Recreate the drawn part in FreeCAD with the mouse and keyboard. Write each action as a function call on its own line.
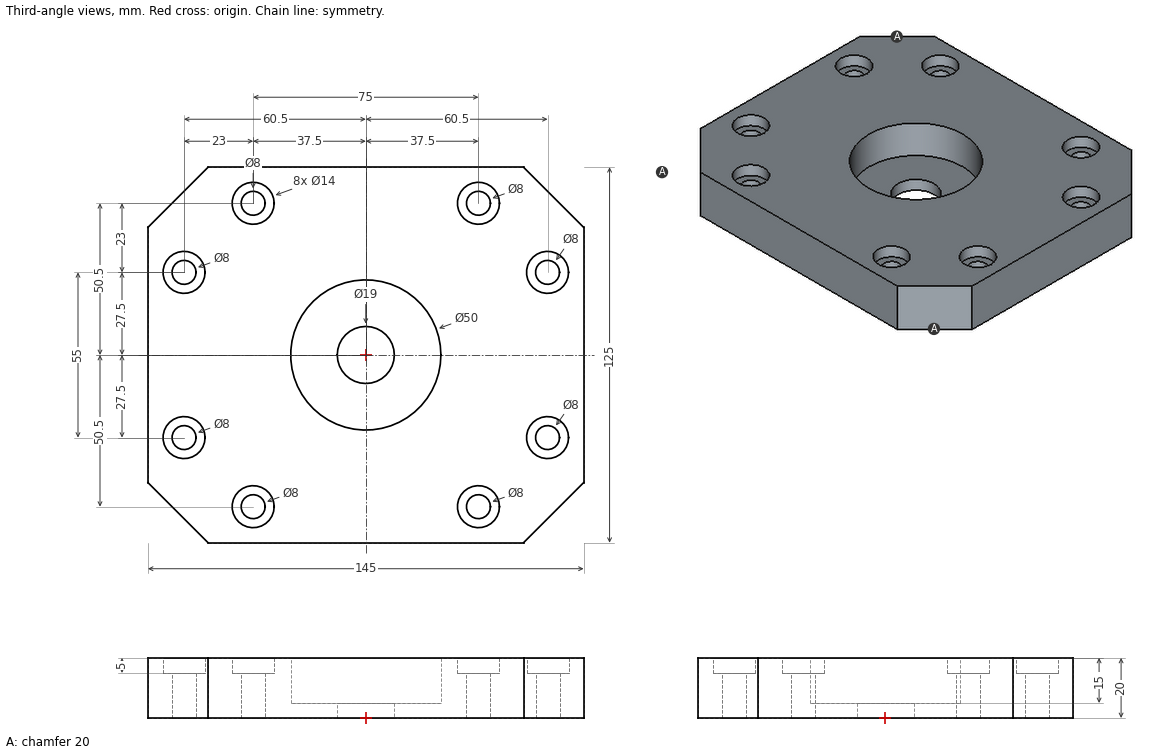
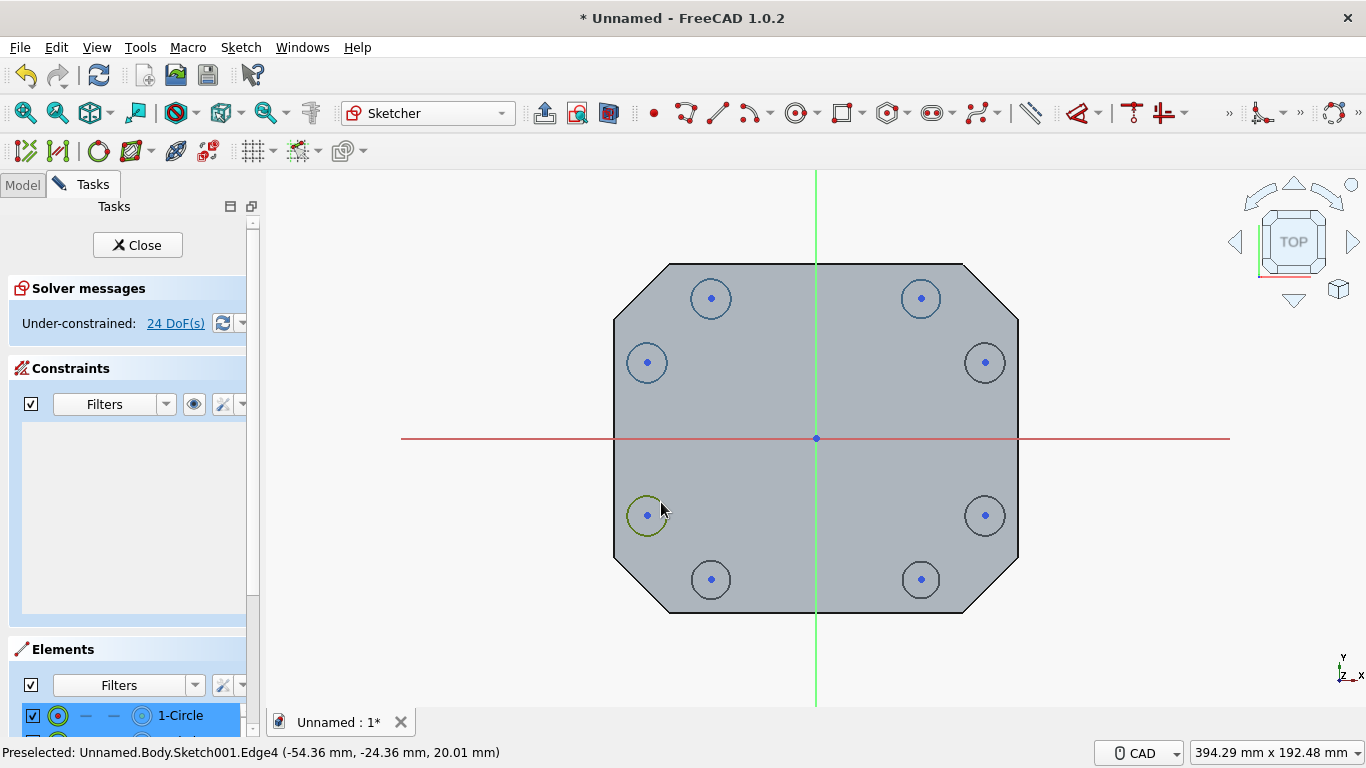
click(724, 566)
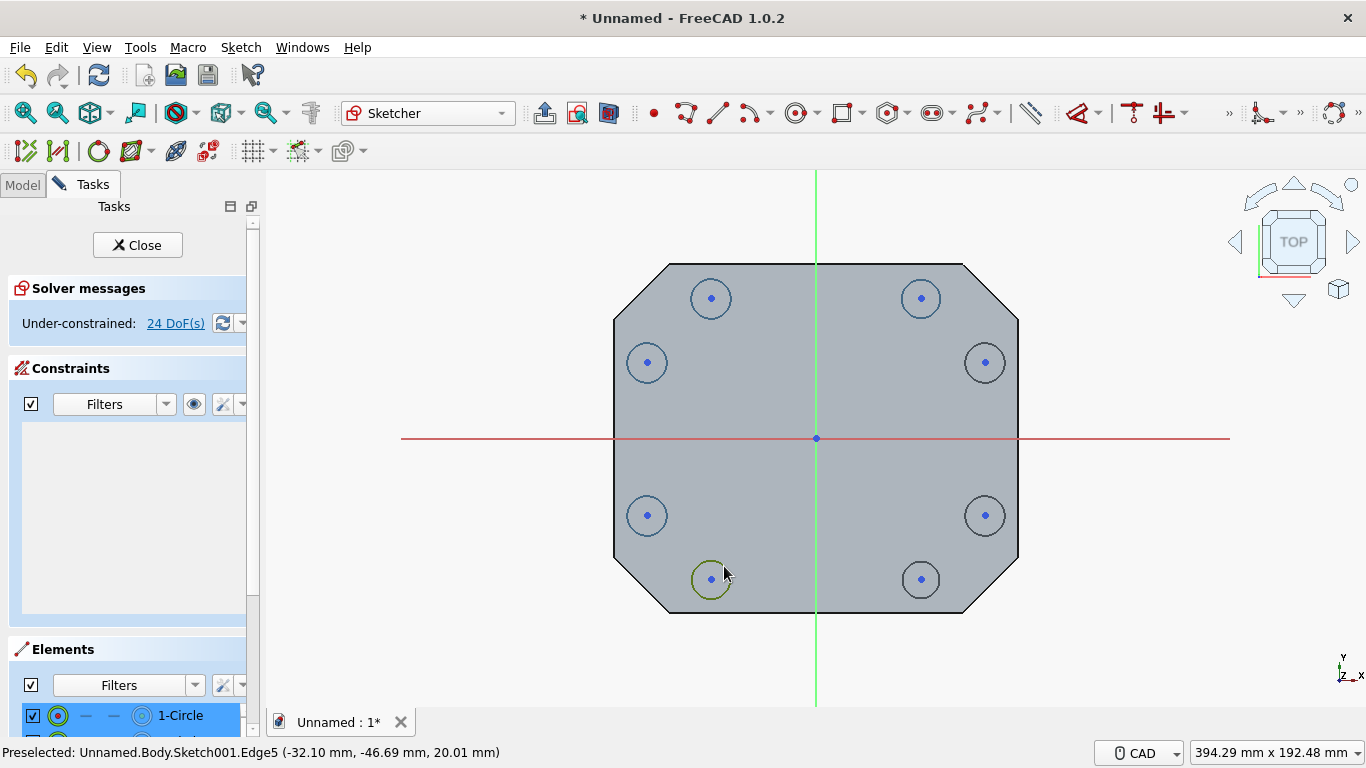
click(934, 567)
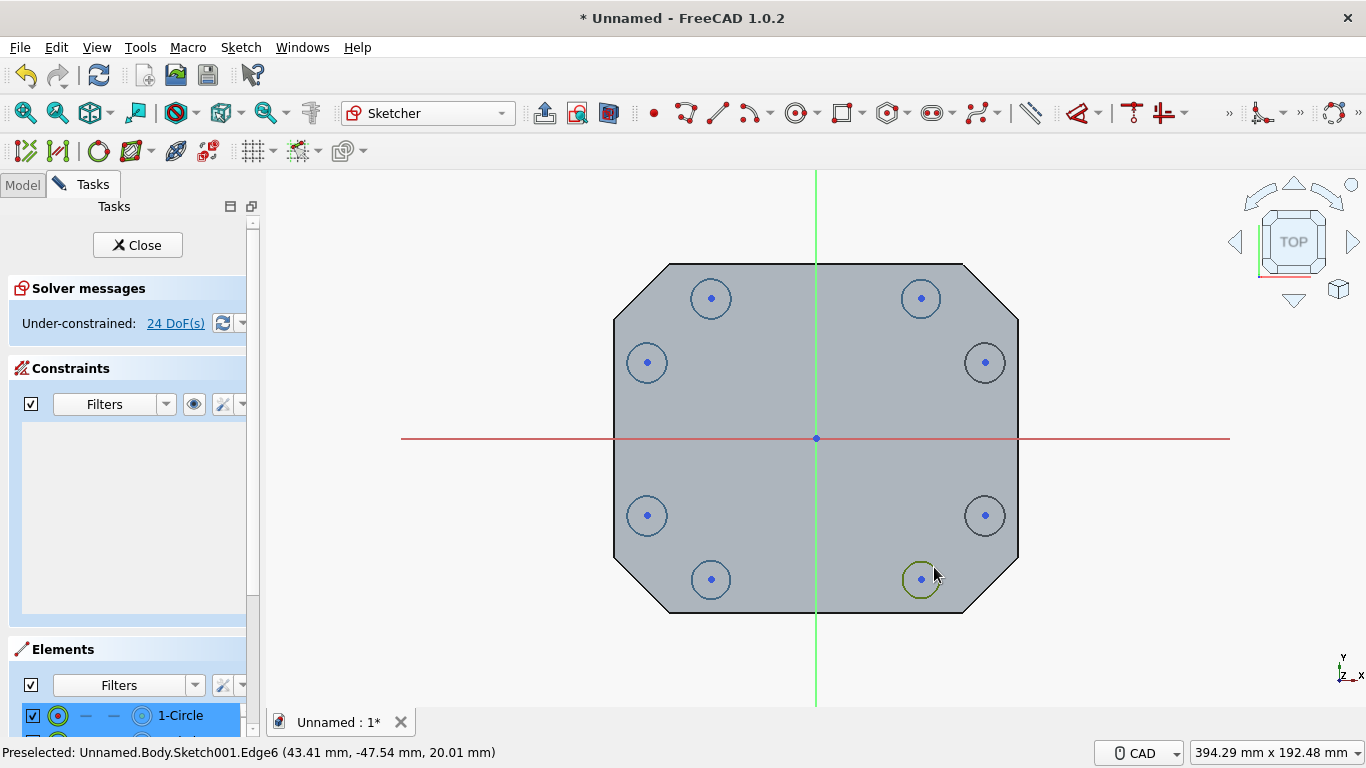
click(999, 349)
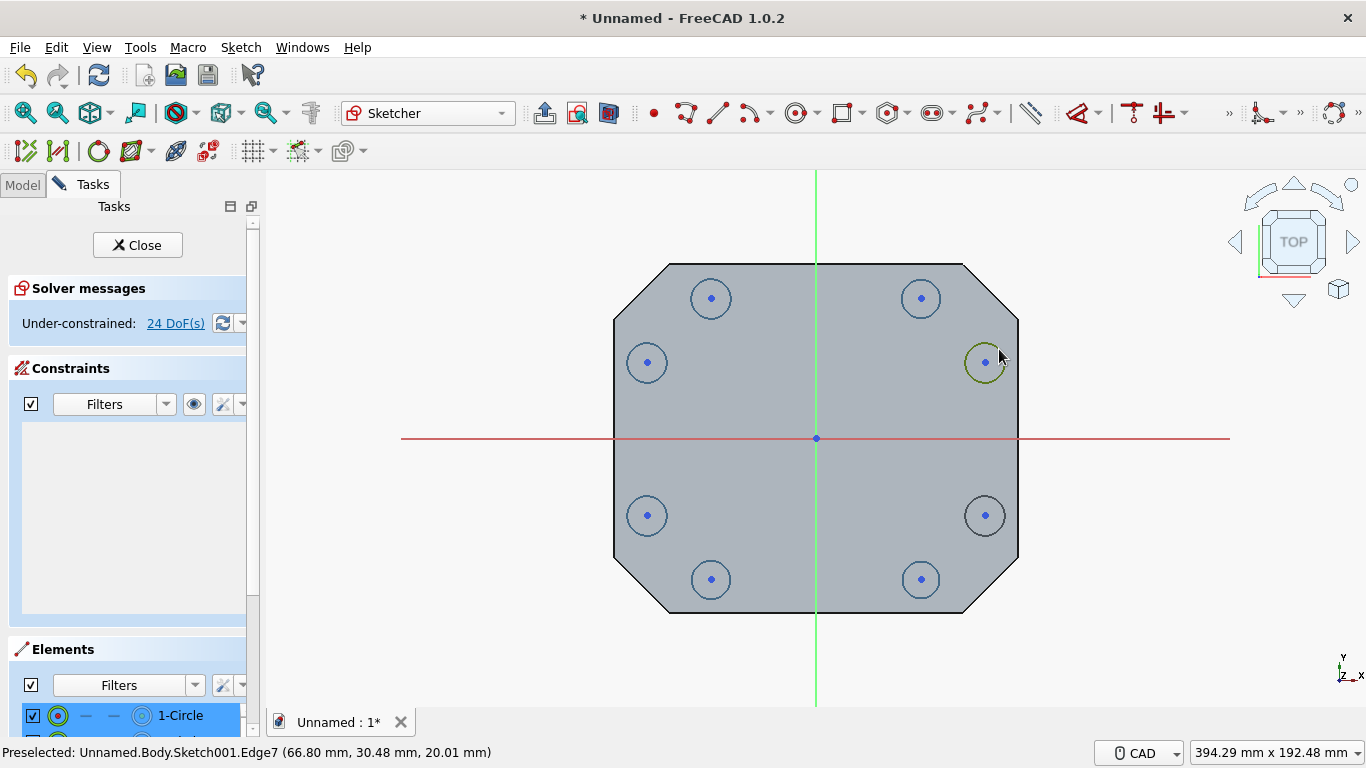
click(999, 502)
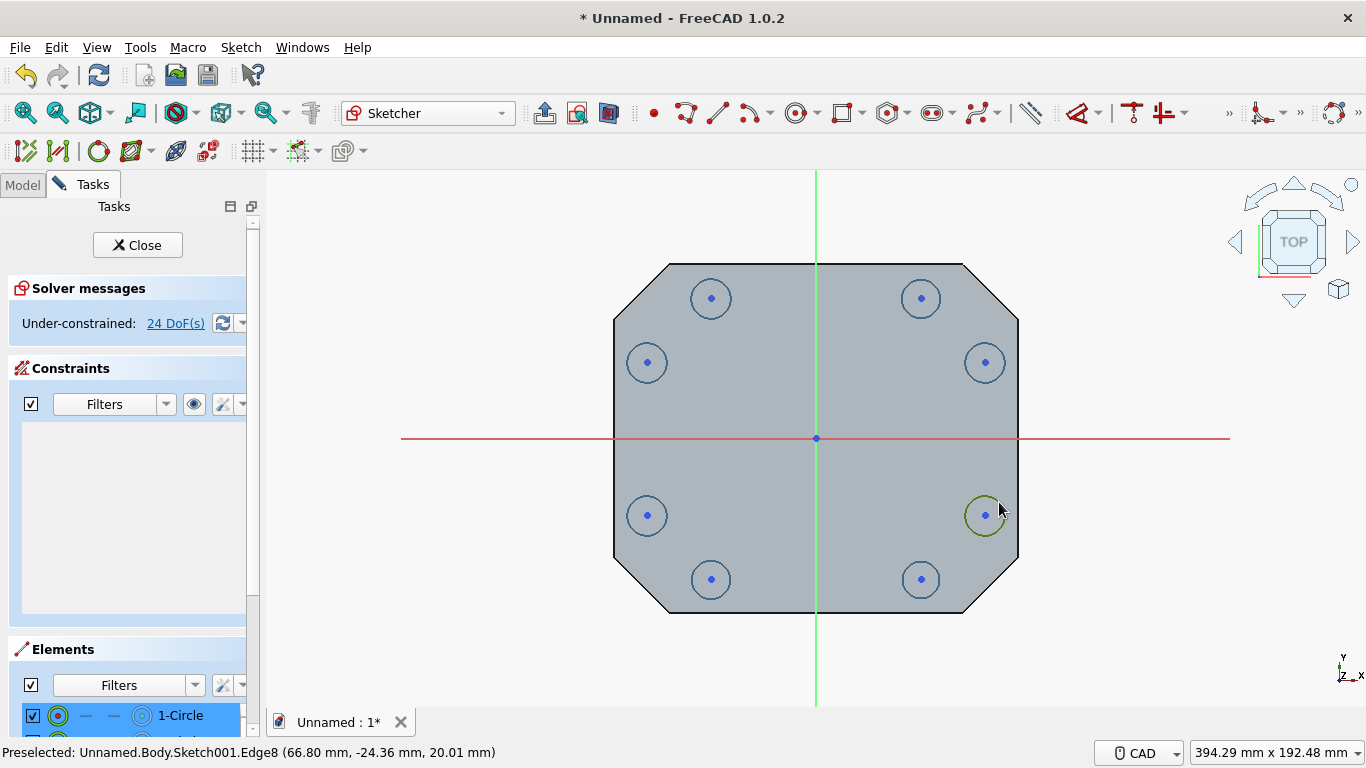
key(e)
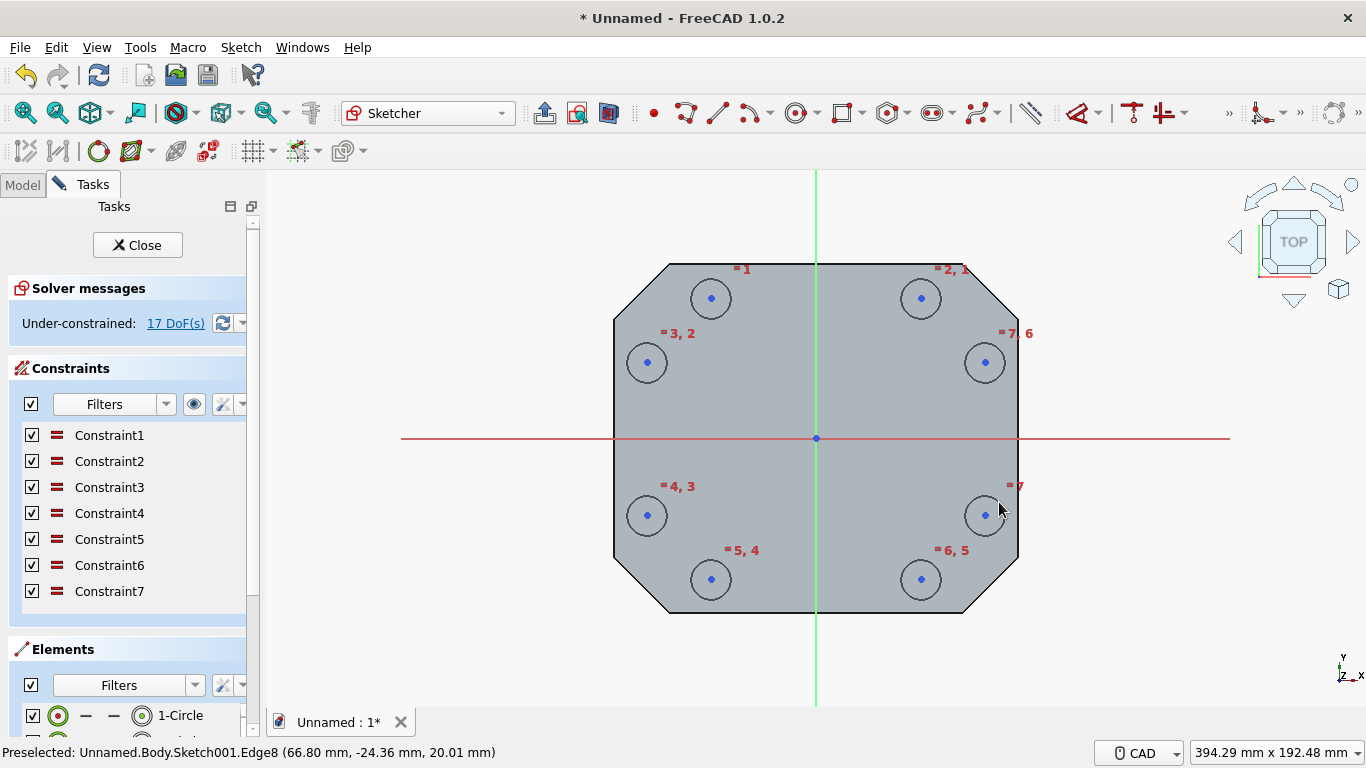
click(711, 299)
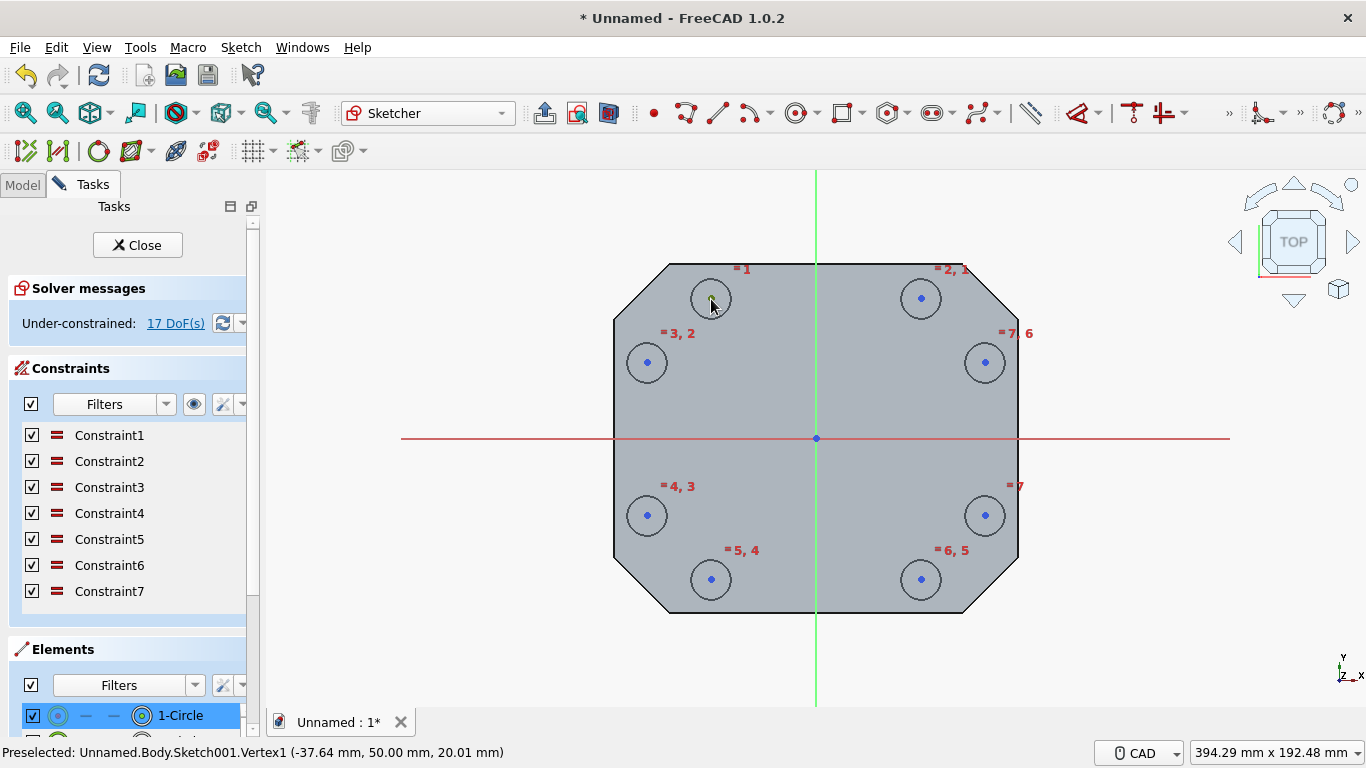
click(921, 299)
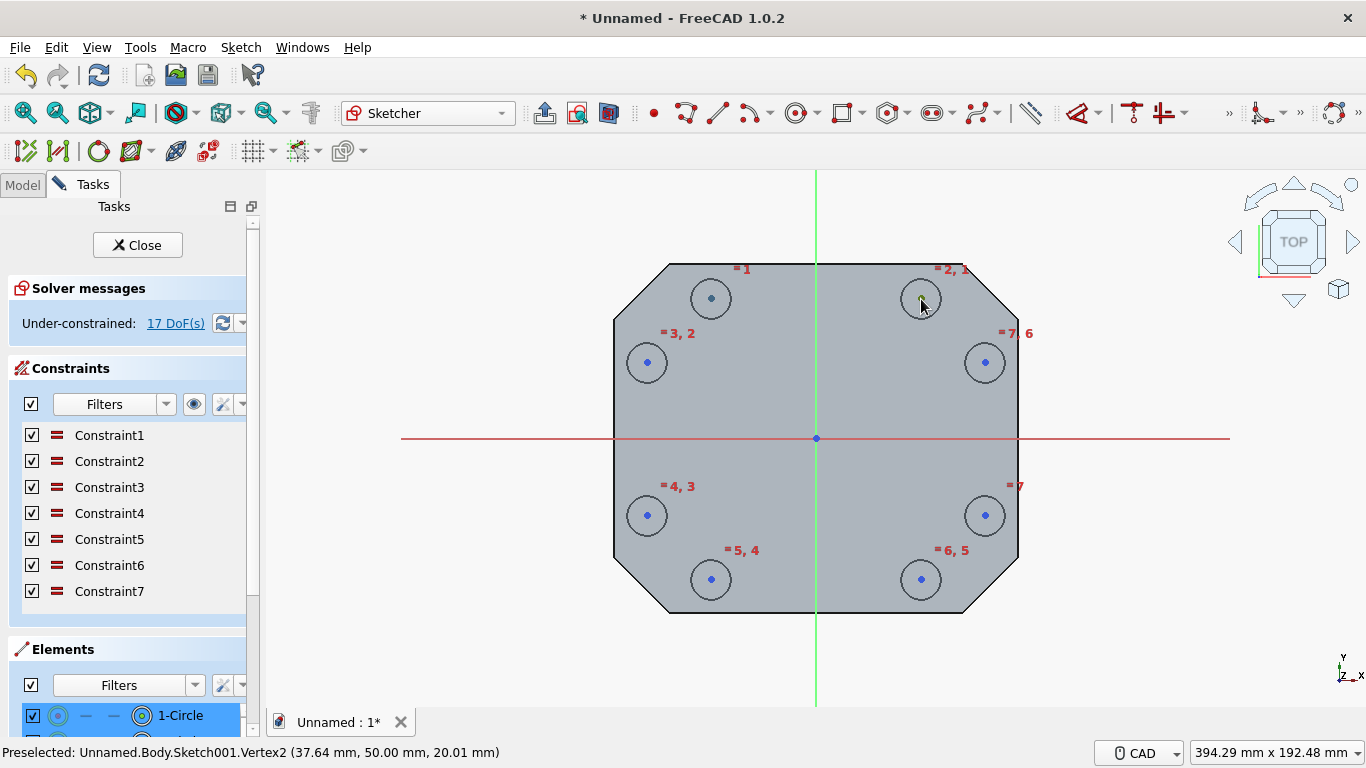
click(816, 645)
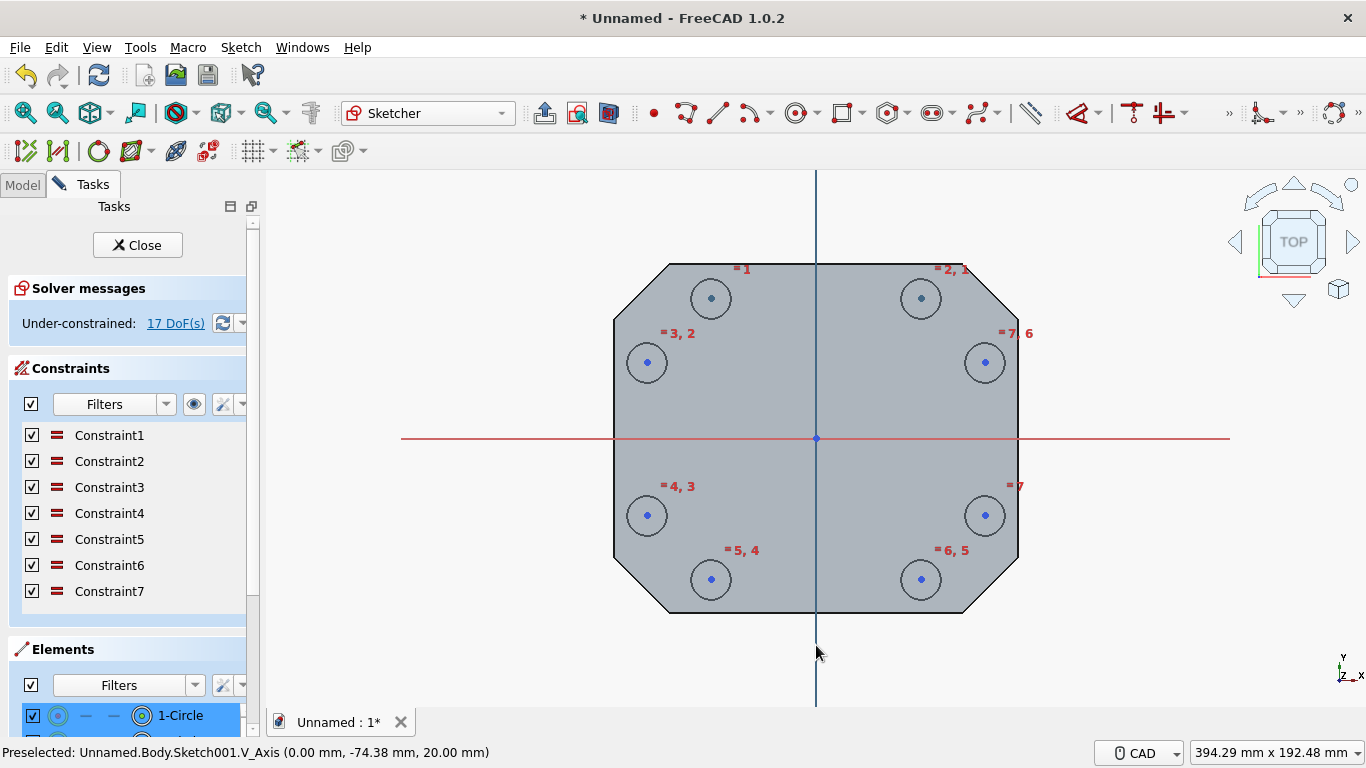
key(s)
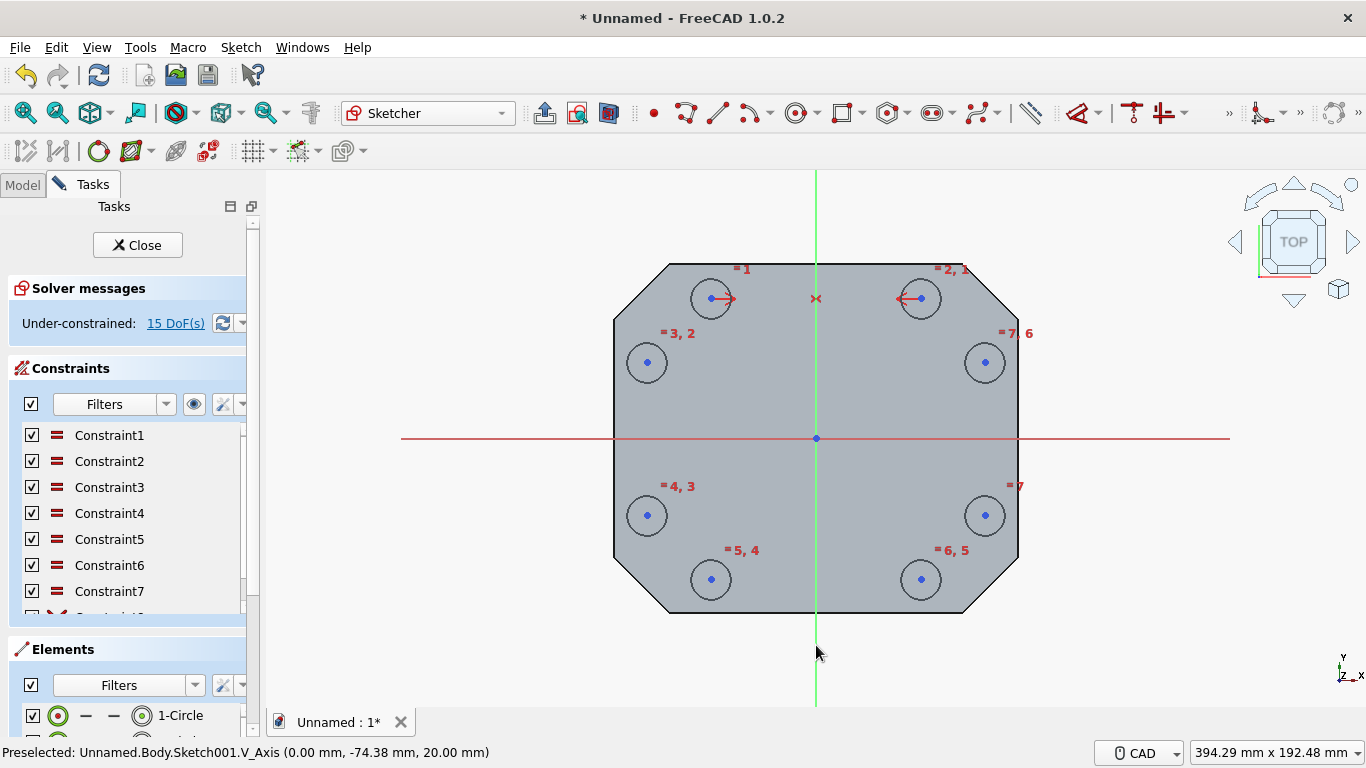
click(647, 363)